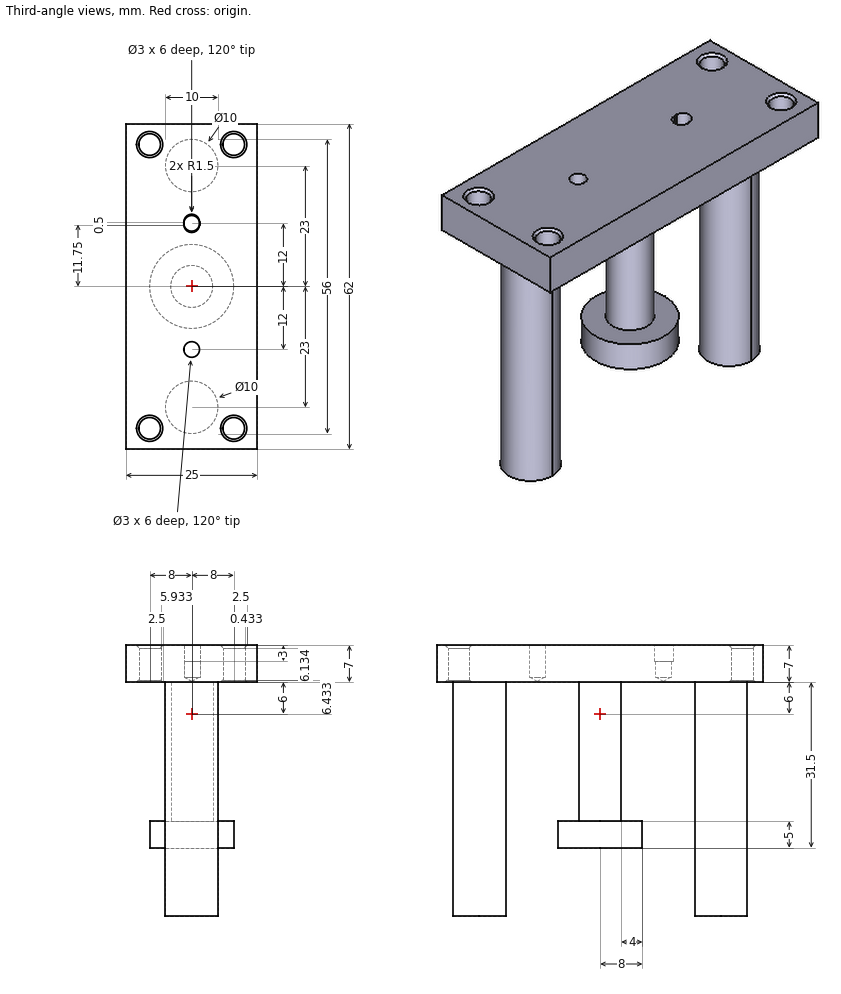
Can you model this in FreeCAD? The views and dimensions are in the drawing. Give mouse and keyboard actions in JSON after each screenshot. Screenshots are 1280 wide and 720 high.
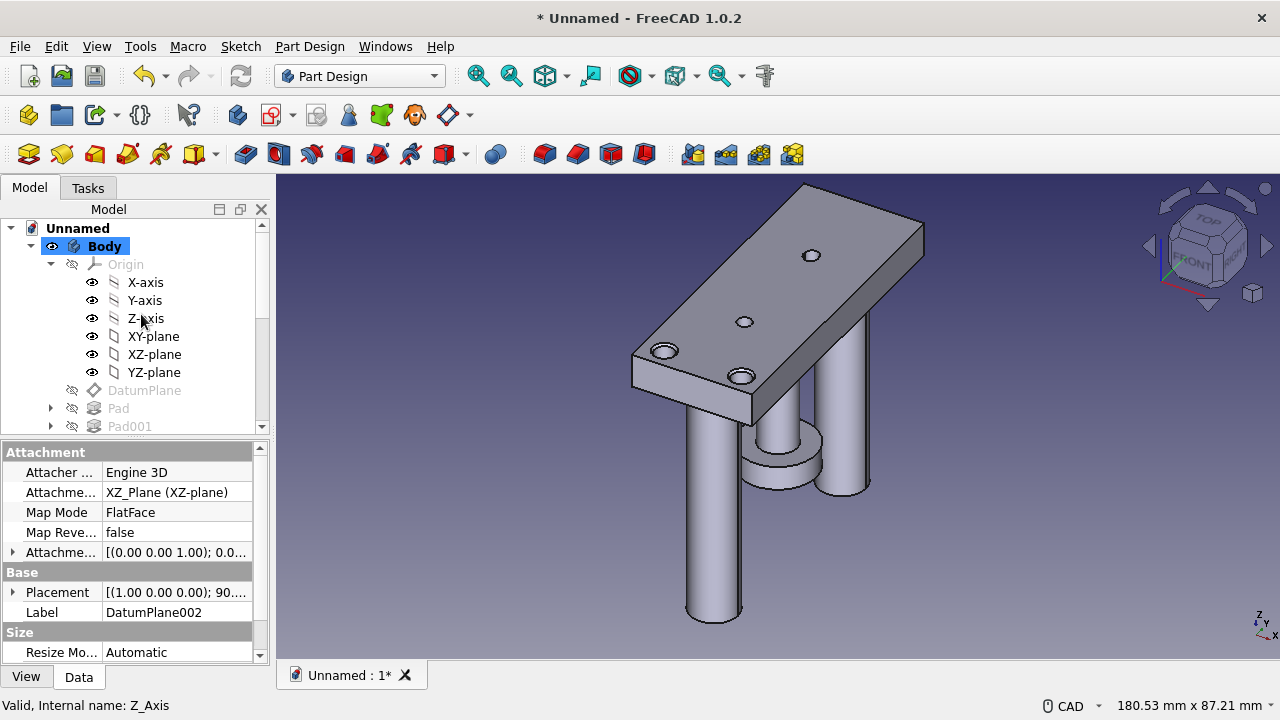
{"action": "left_click", "coordinate": [137, 354]}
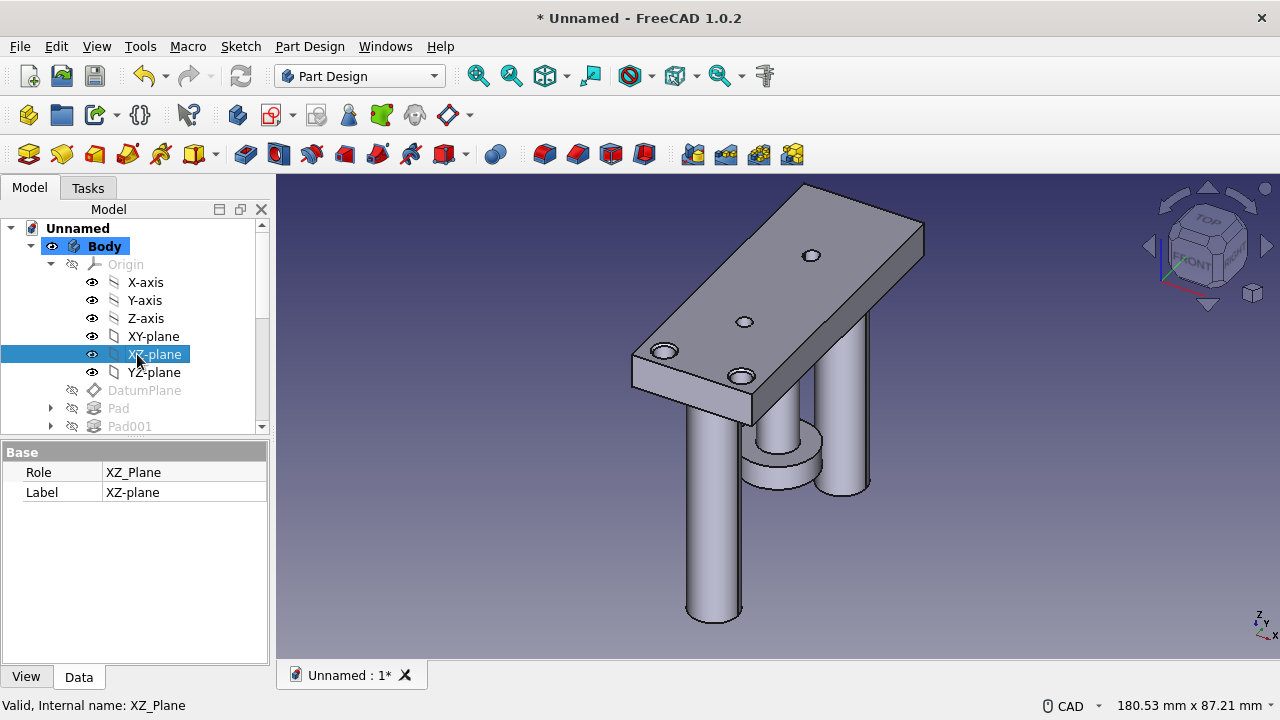
{"action": "left_click", "coordinate": [448, 116]}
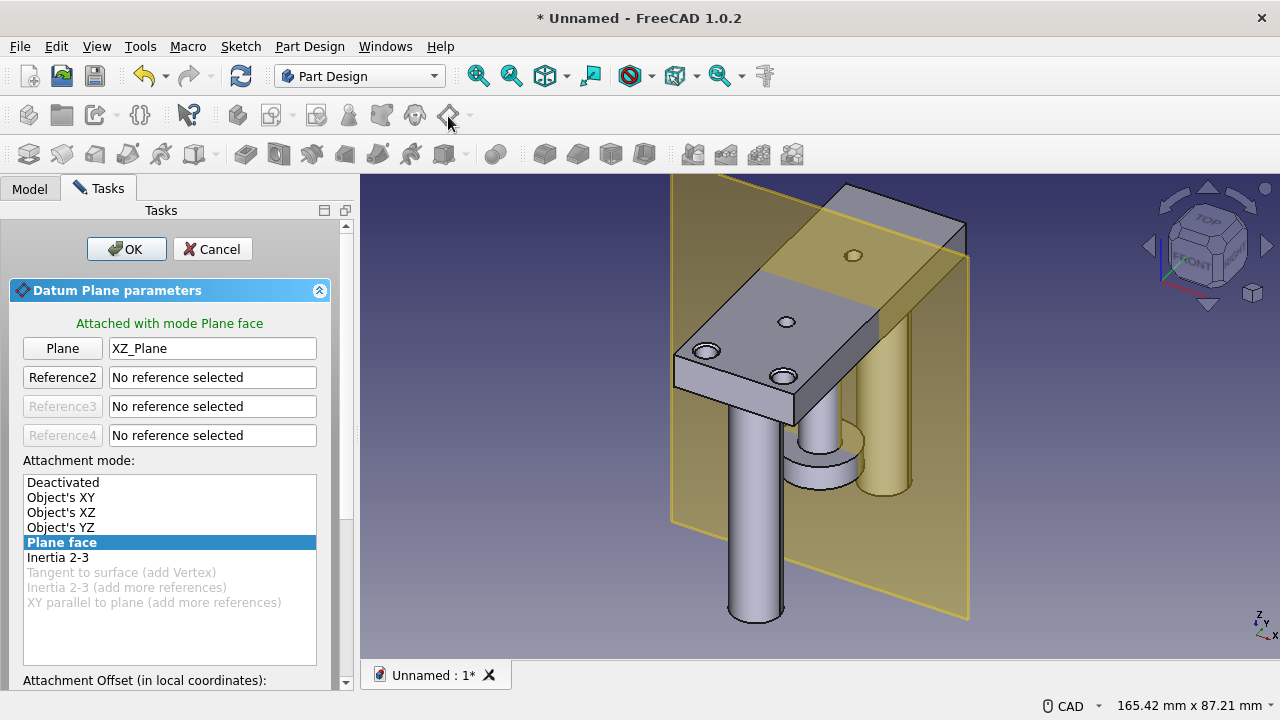
{"action": "scroll", "coordinate": [346, 455], "scroll_direction": "down", "scroll_amount": 3}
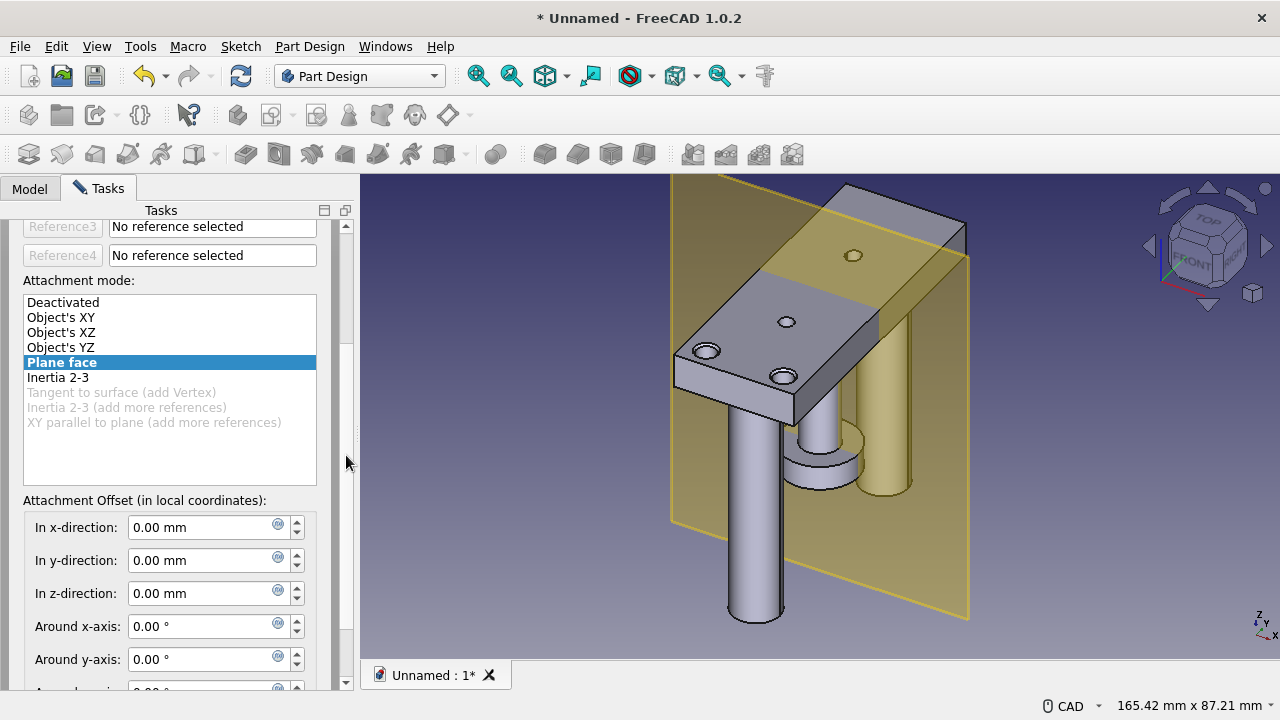
{"action": "triple_click", "coordinate": [210, 594]}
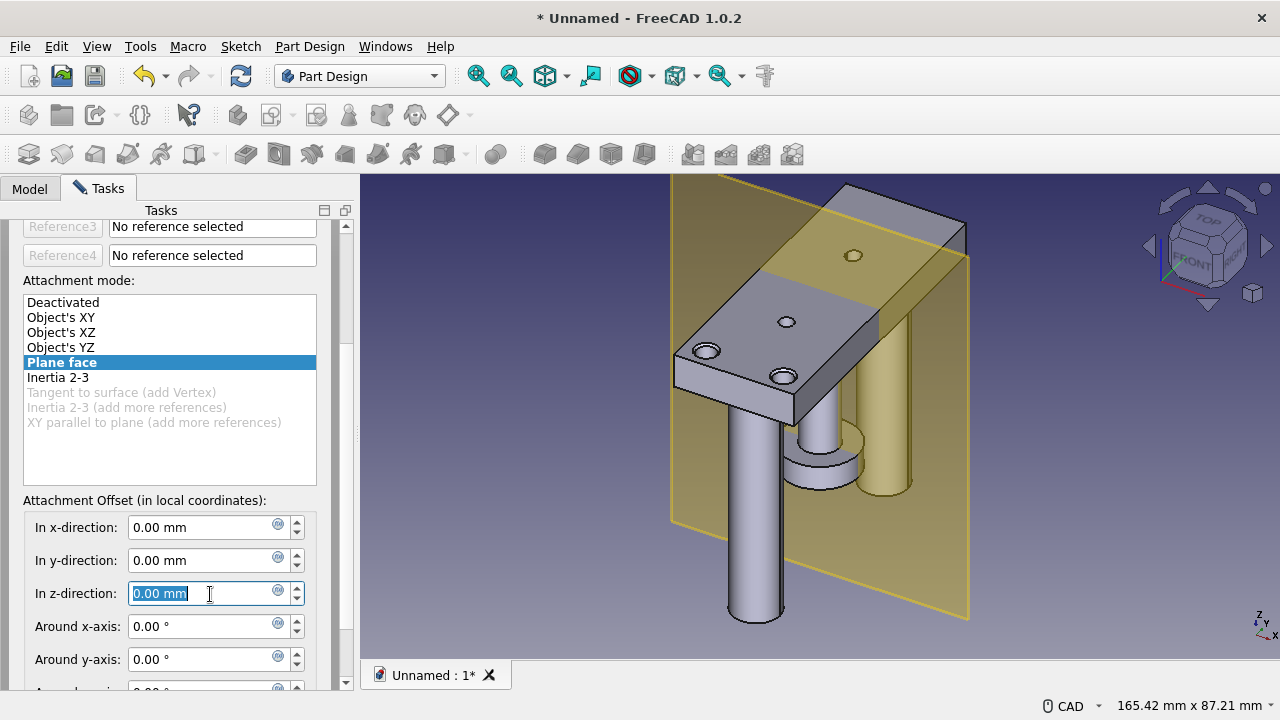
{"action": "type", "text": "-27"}
{"action": "key", "text": "Tab"}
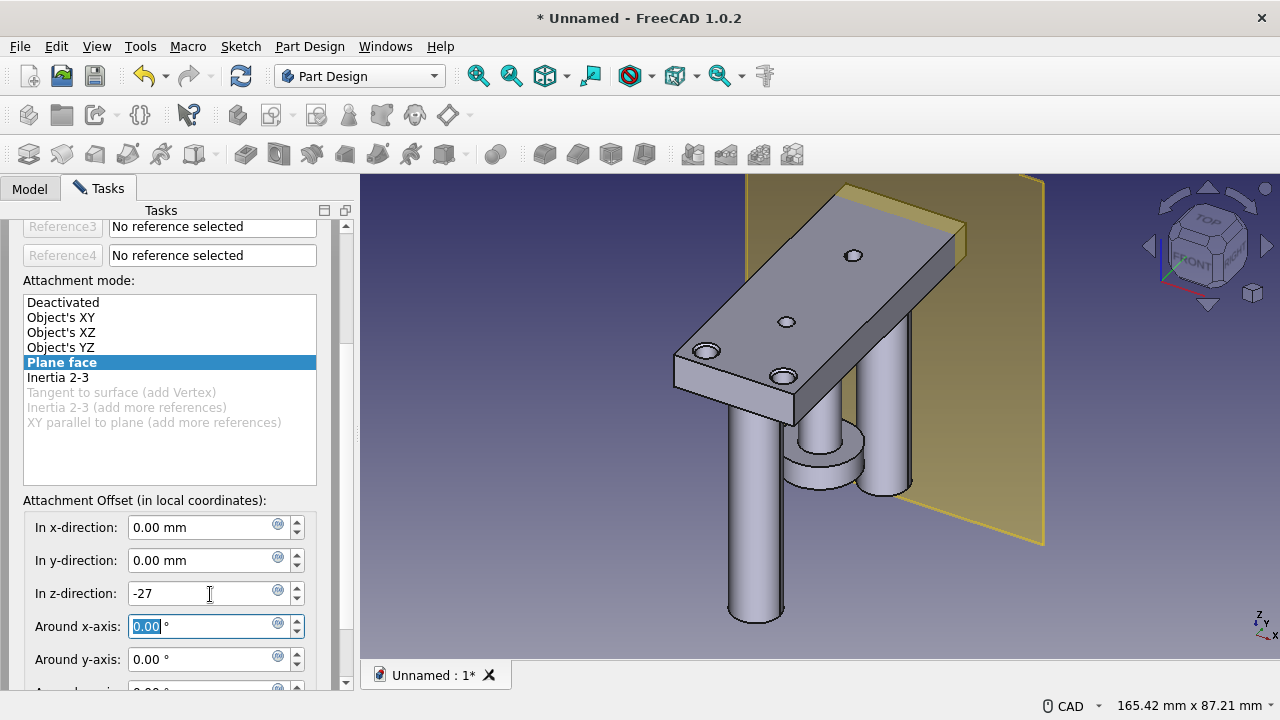
{"action": "scroll", "coordinate": [346, 455], "scroll_direction": "up", "scroll_amount": 4}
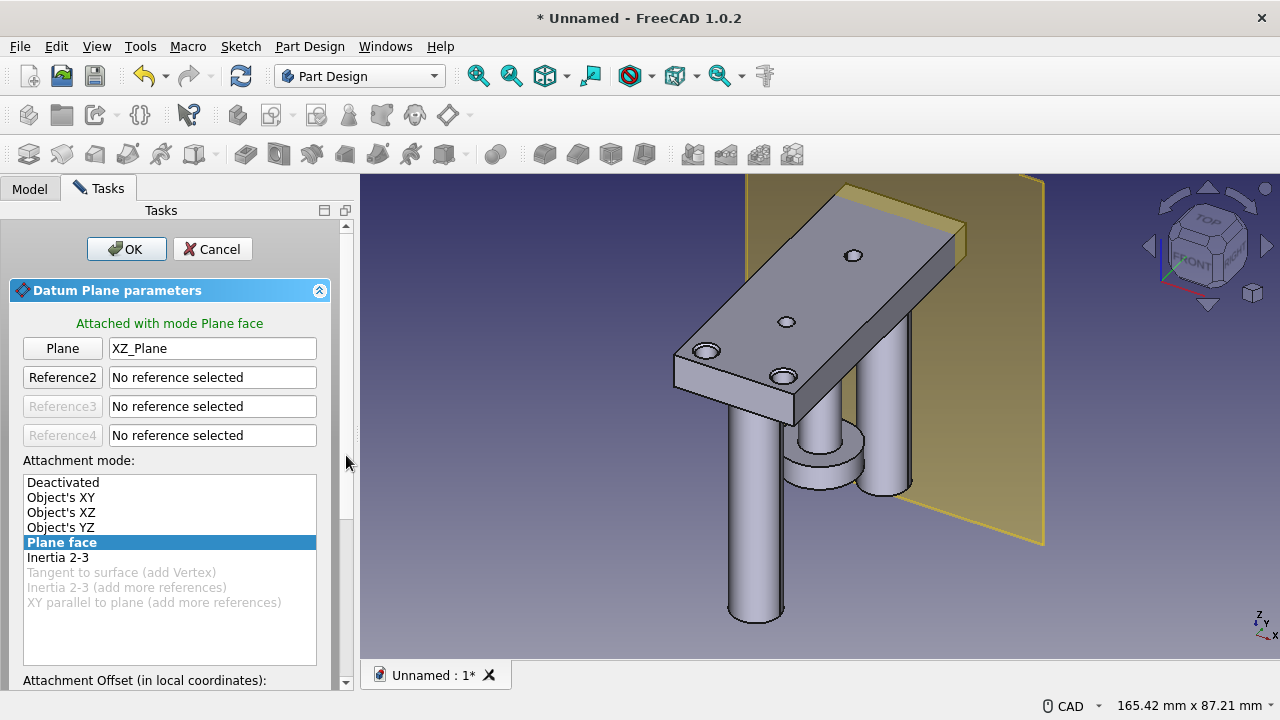
{"action": "left_click", "coordinate": [127, 249]}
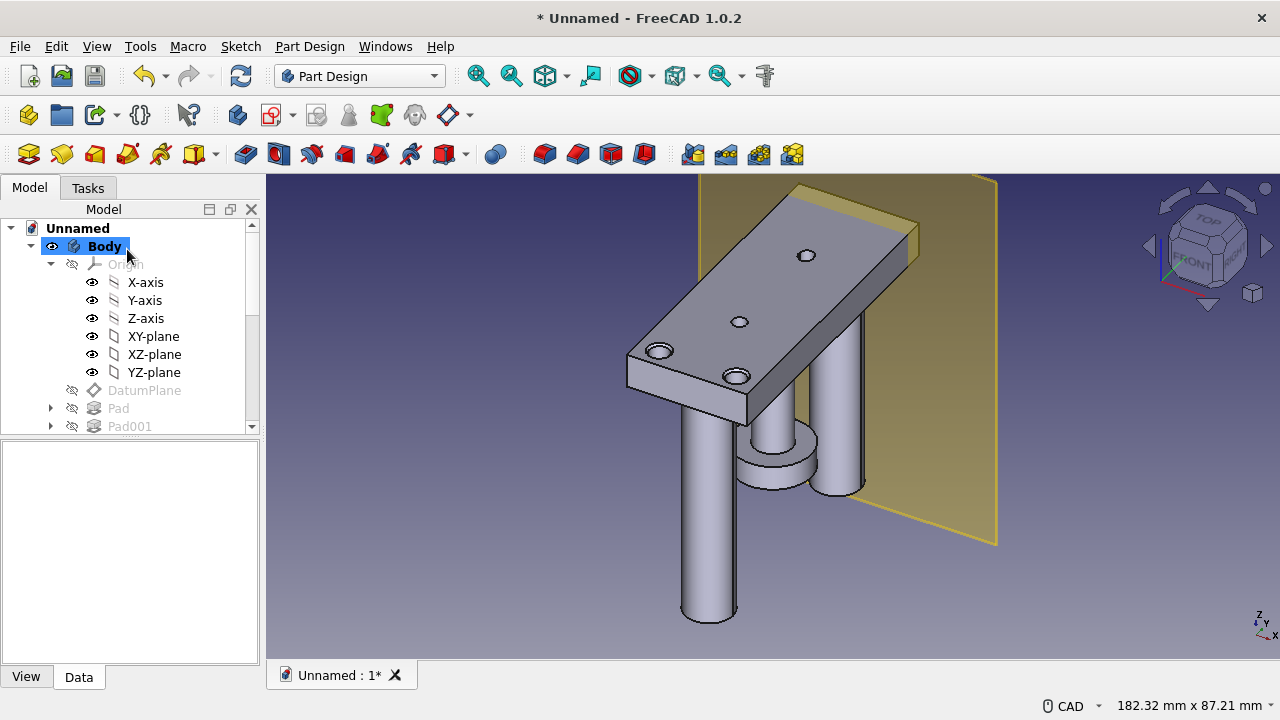
{"action": "scroll", "coordinate": [101, 332], "scroll_direction": "down", "scroll_amount": 3}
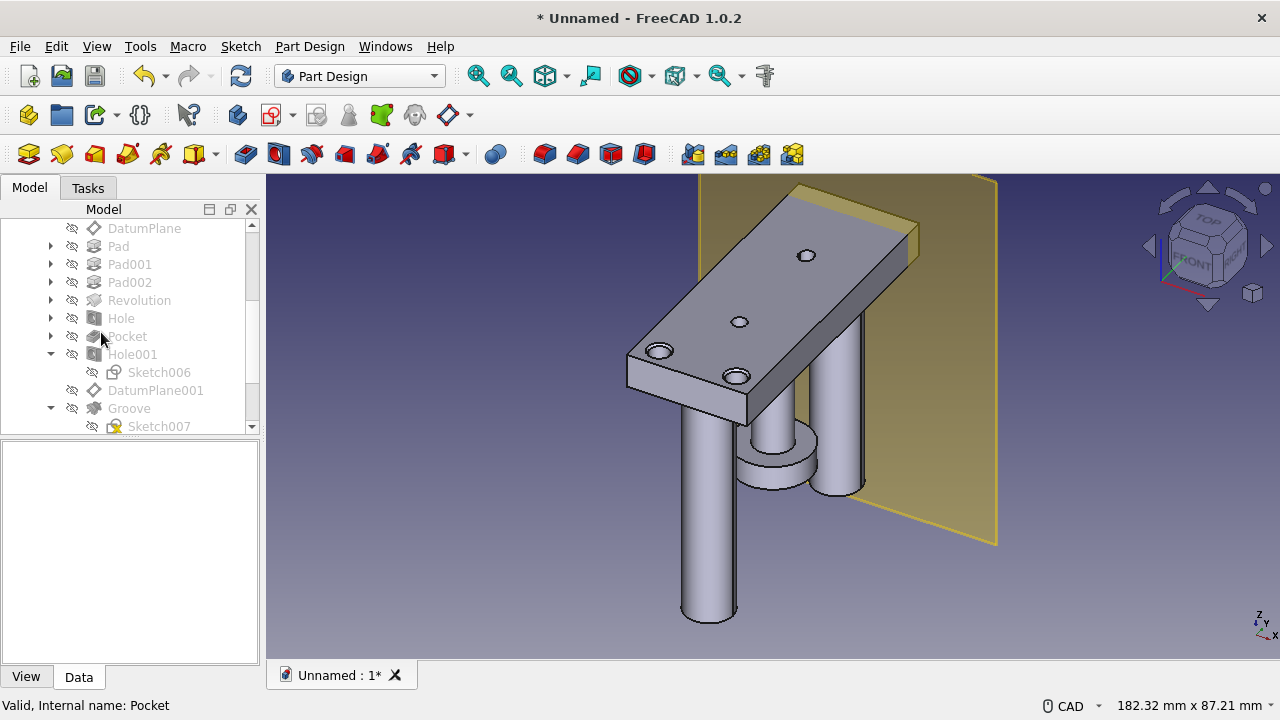
{"action": "scroll", "coordinate": [141, 332], "scroll_direction": "up", "scroll_amount": 15}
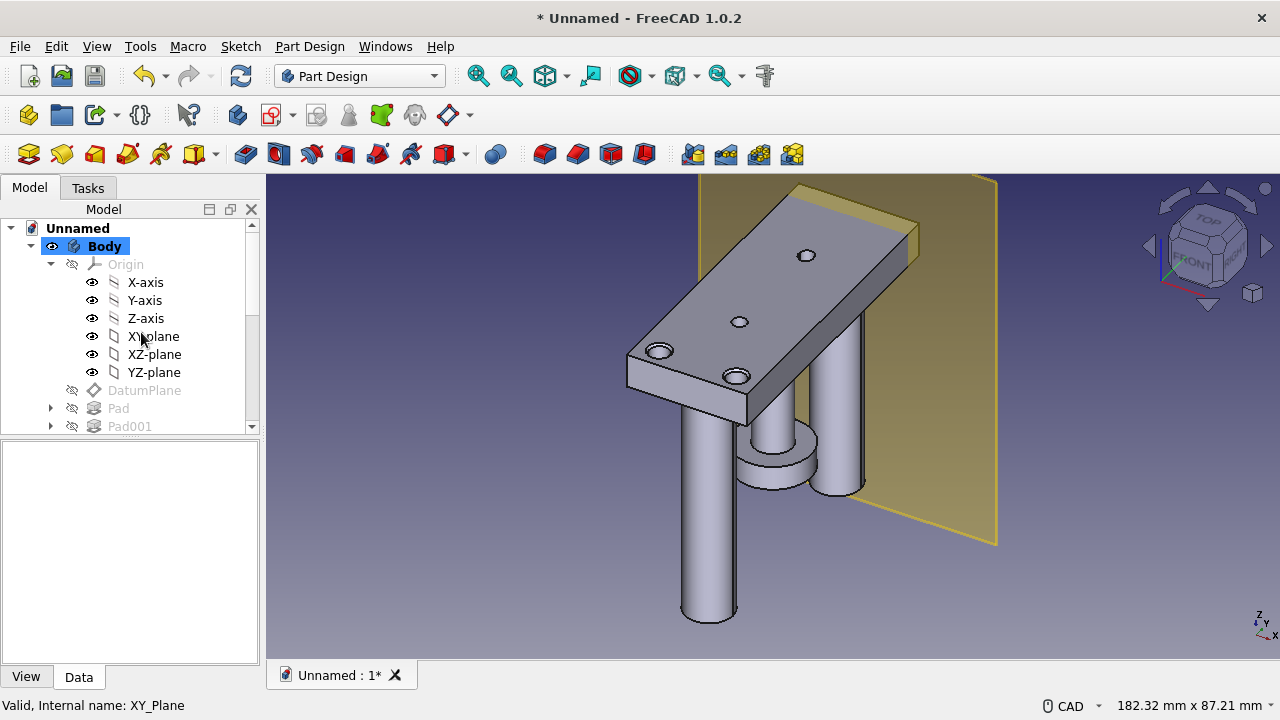
{"action": "scroll", "coordinate": [101, 332], "scroll_direction": "down", "scroll_amount": 6}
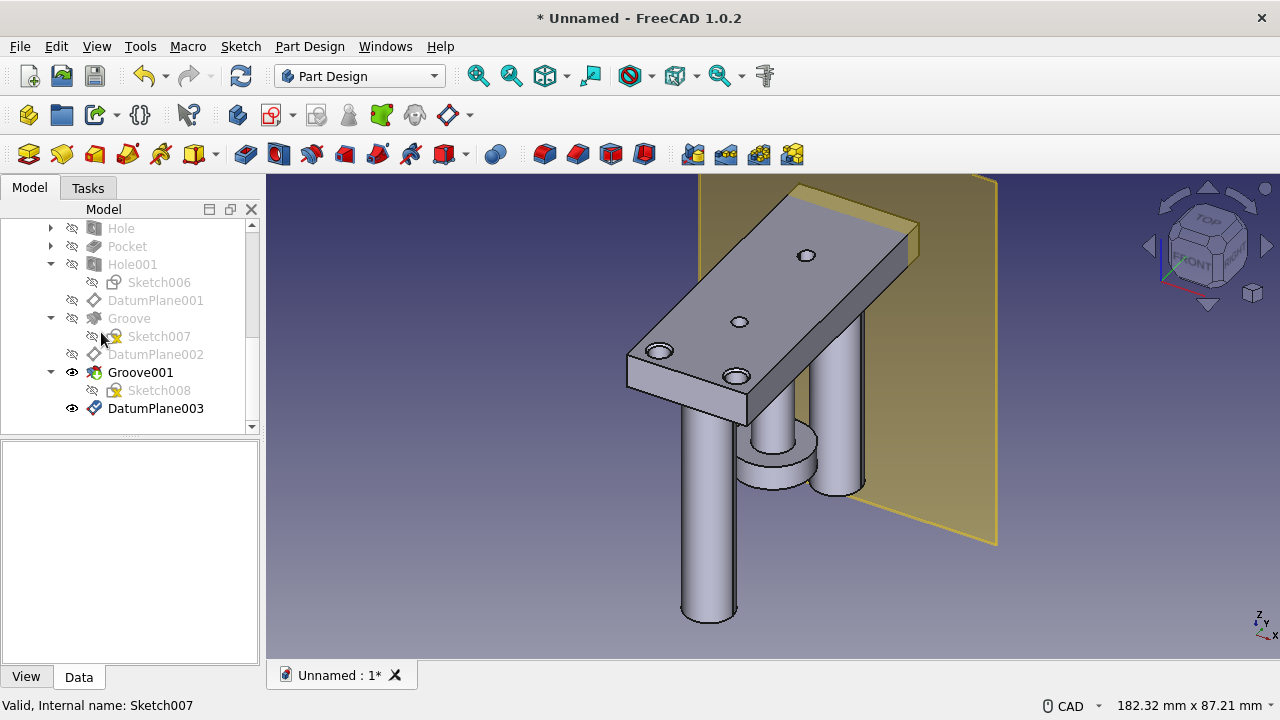
{"action": "left_click", "coordinate": [117, 408]}